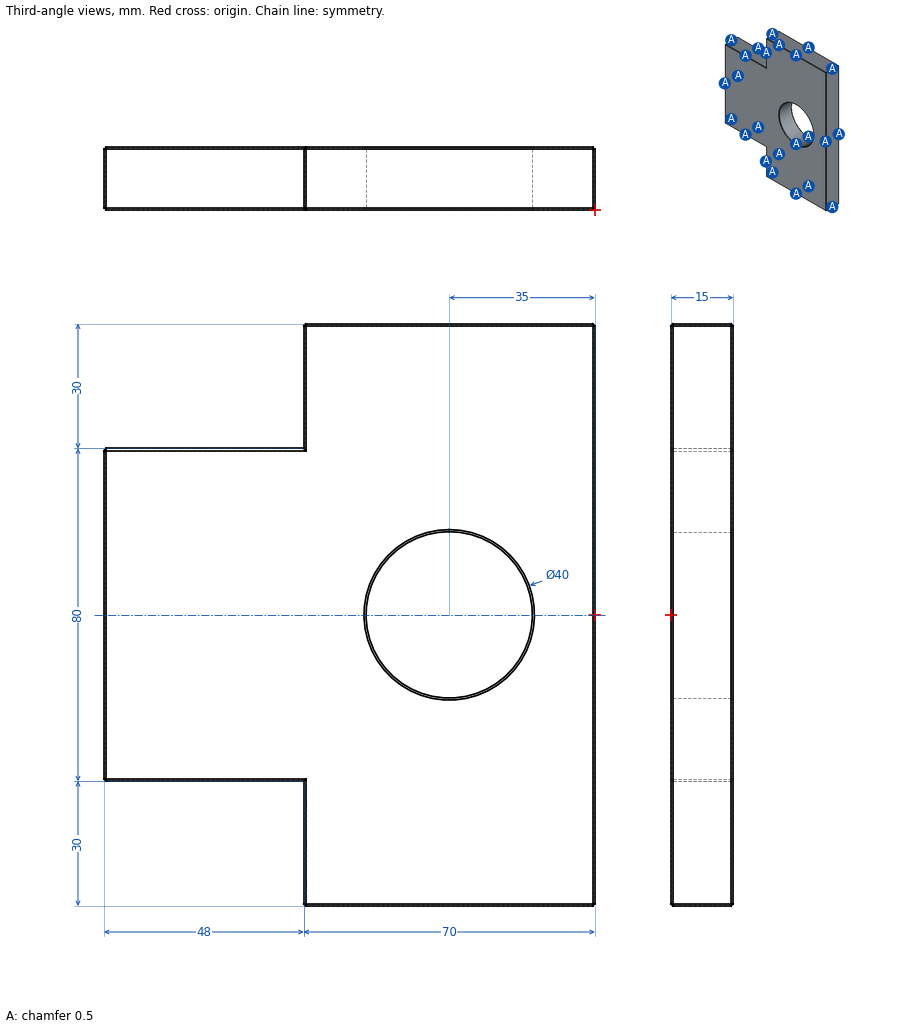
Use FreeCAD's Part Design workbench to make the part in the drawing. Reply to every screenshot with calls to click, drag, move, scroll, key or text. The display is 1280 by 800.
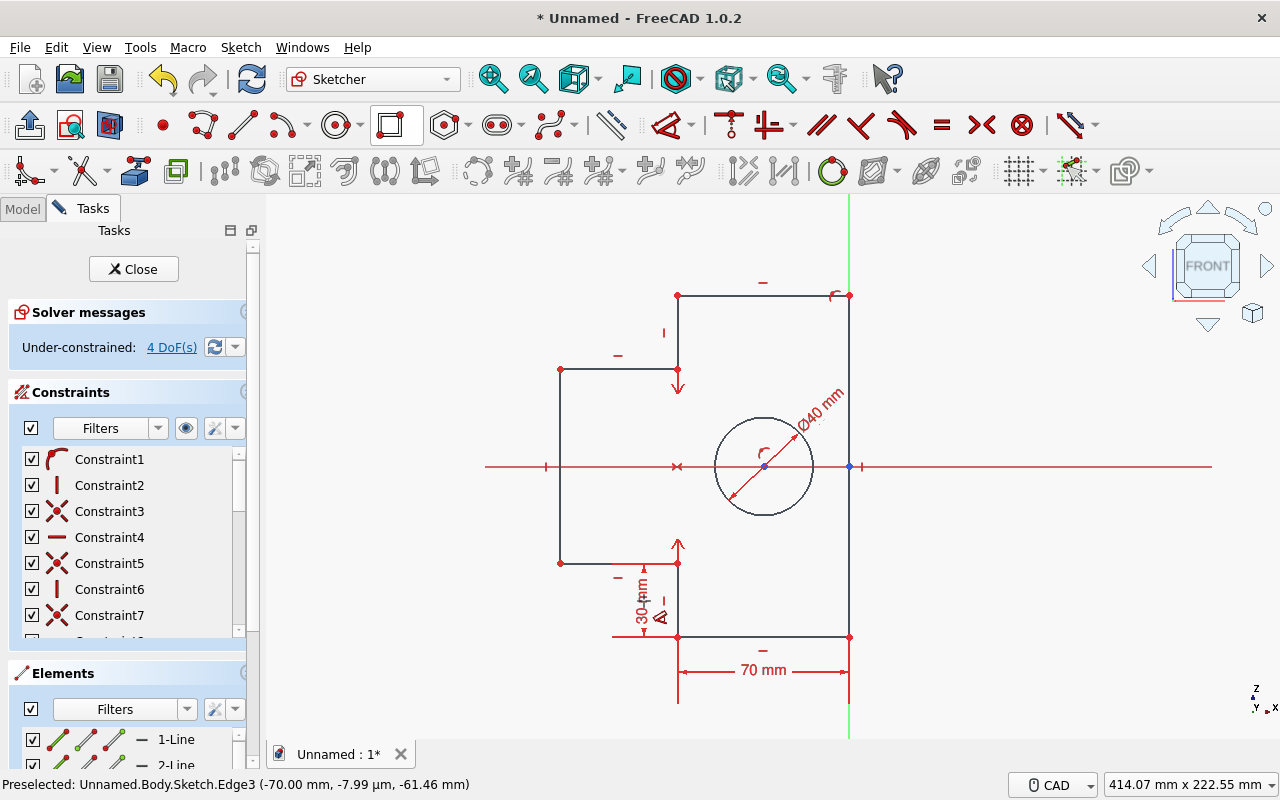
click(643, 564)
click(619, 530)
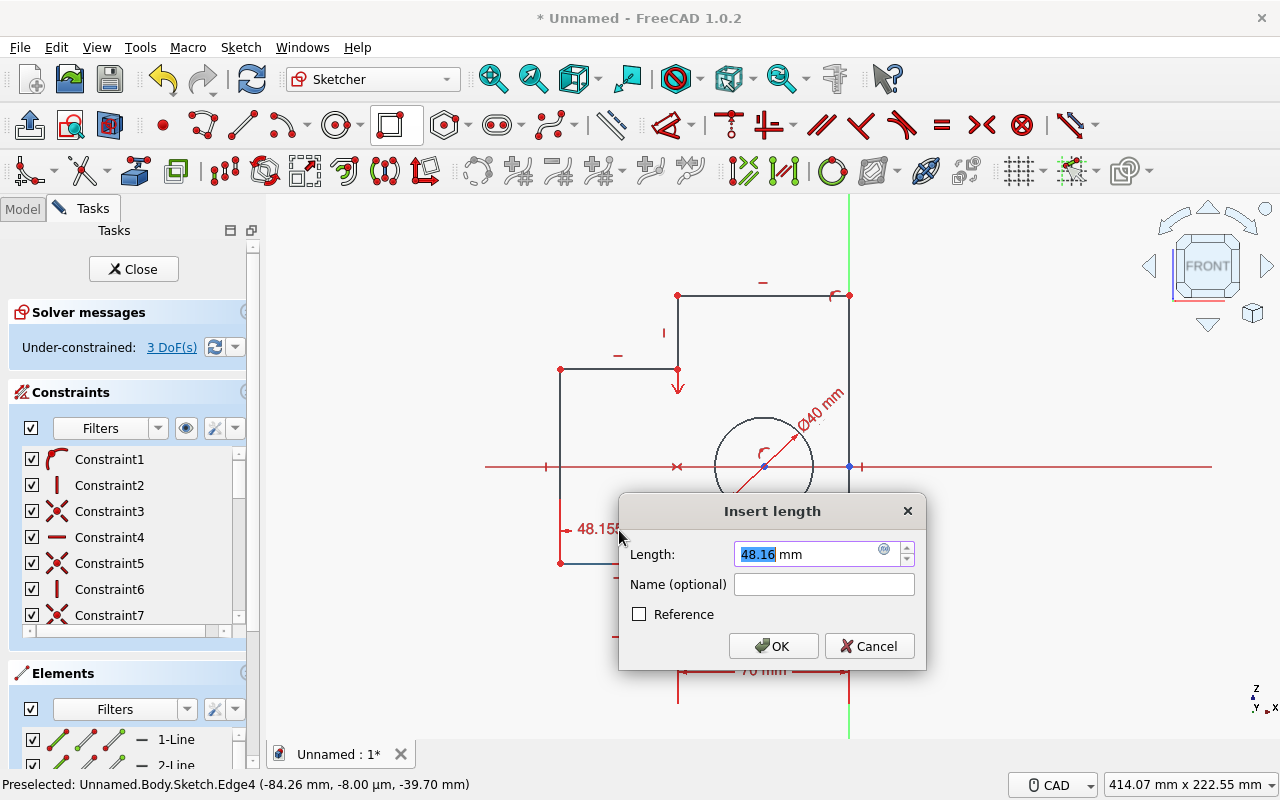
text(48)
key(Return)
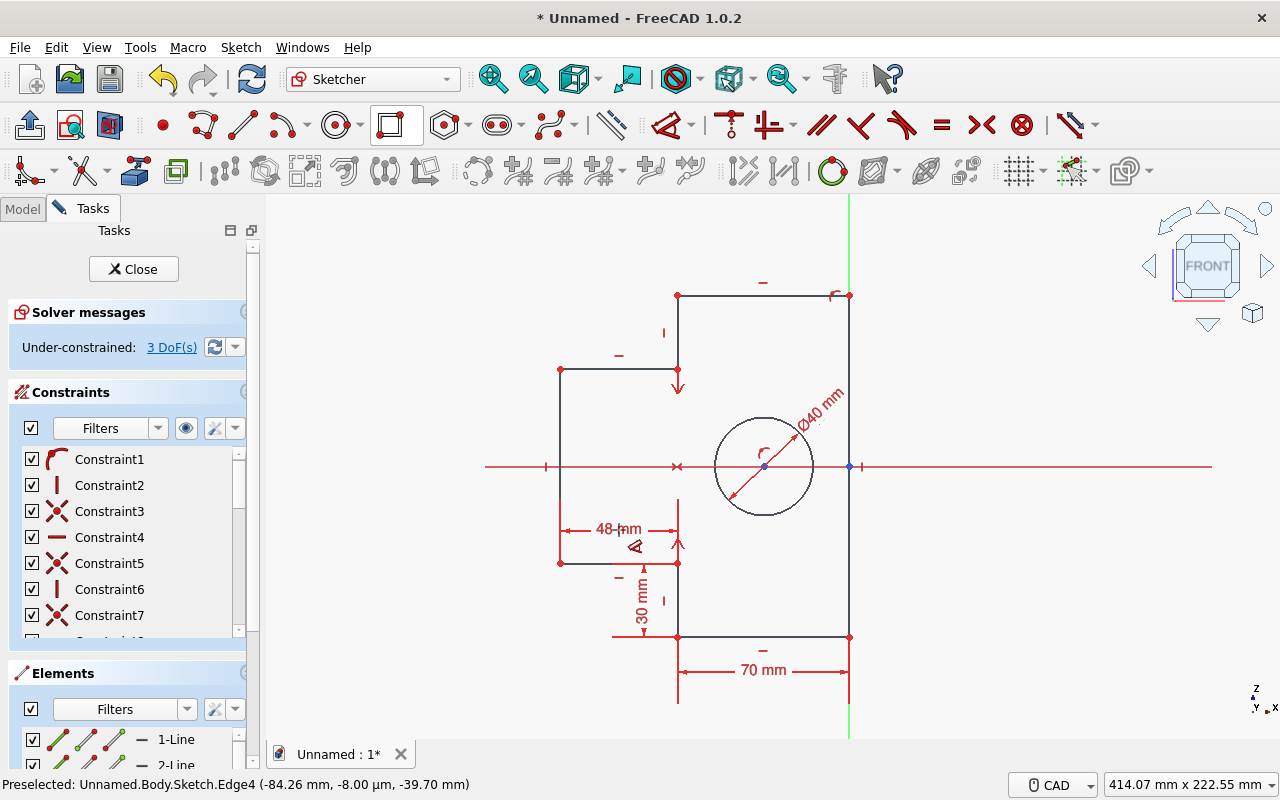
click(560, 505)
click(526, 422)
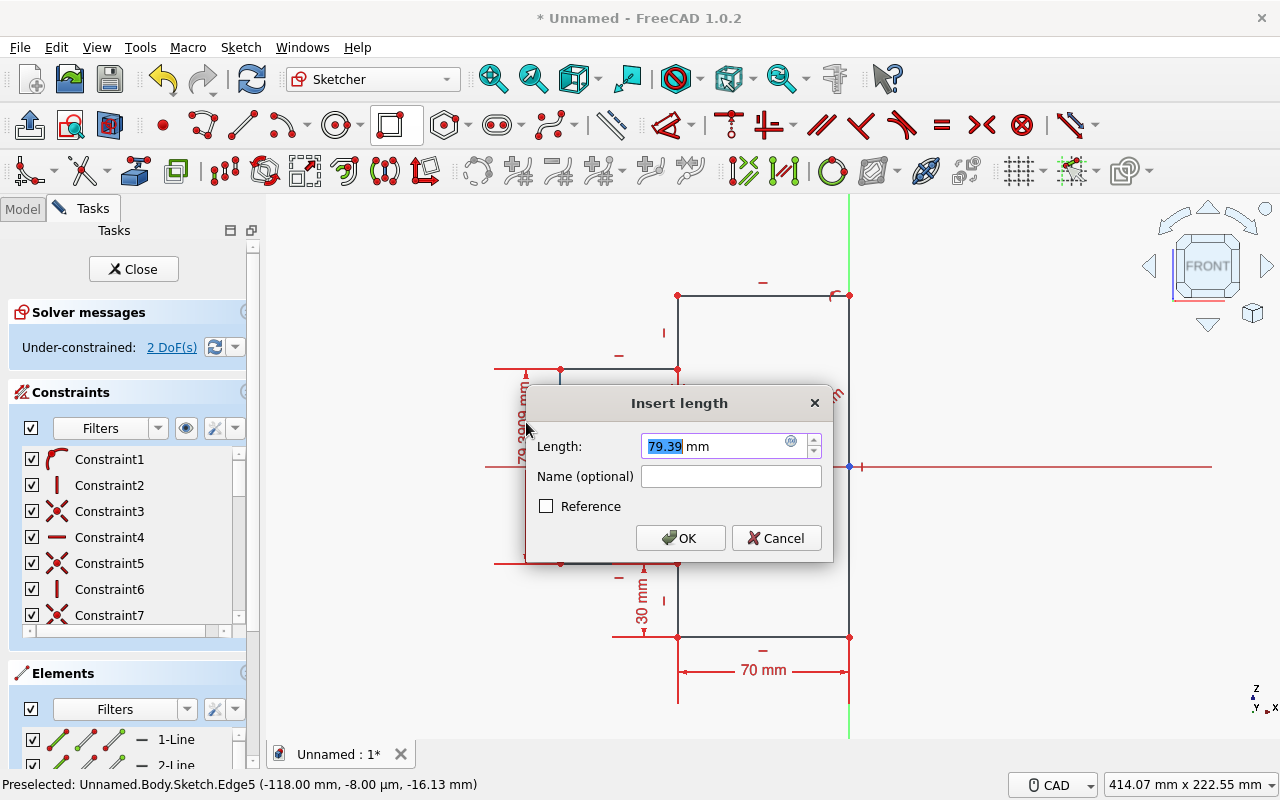
text(80)
key(Return)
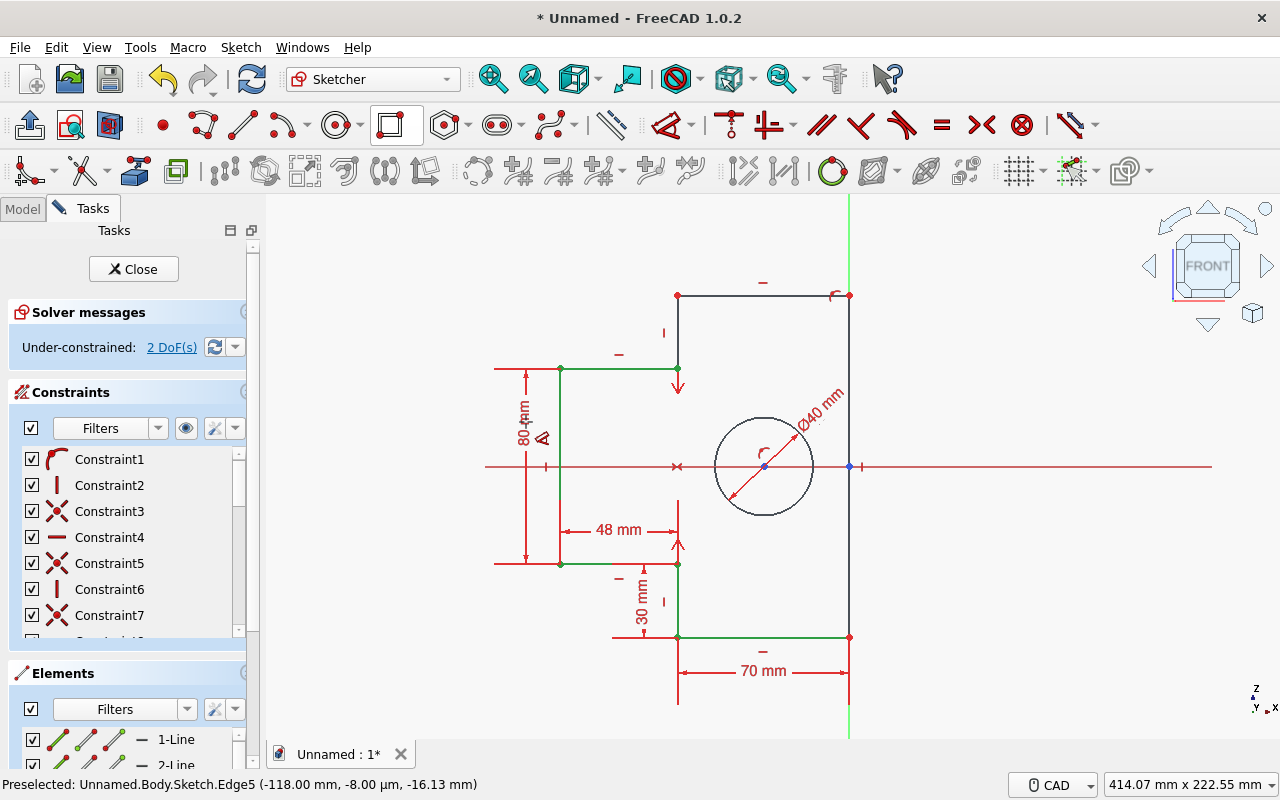
click(678, 347)
click(644, 332)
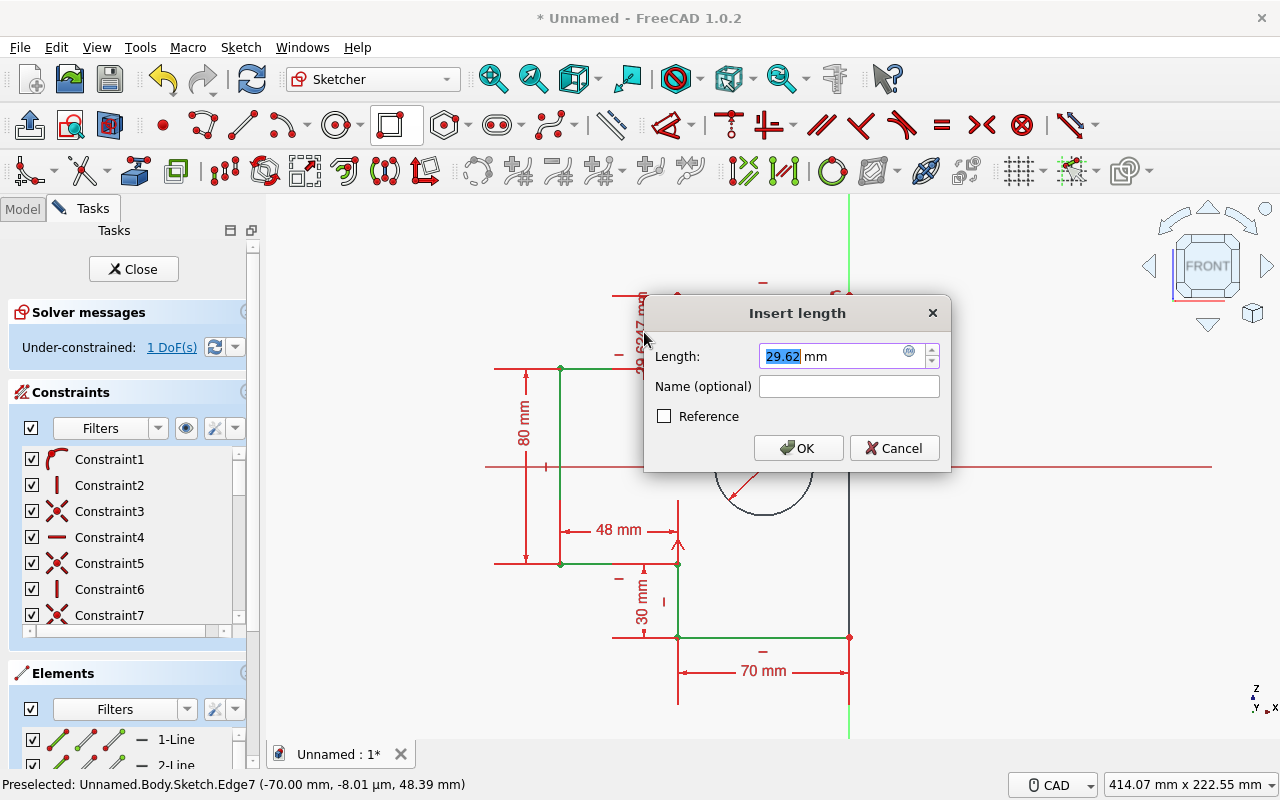
text(30)
key(Return)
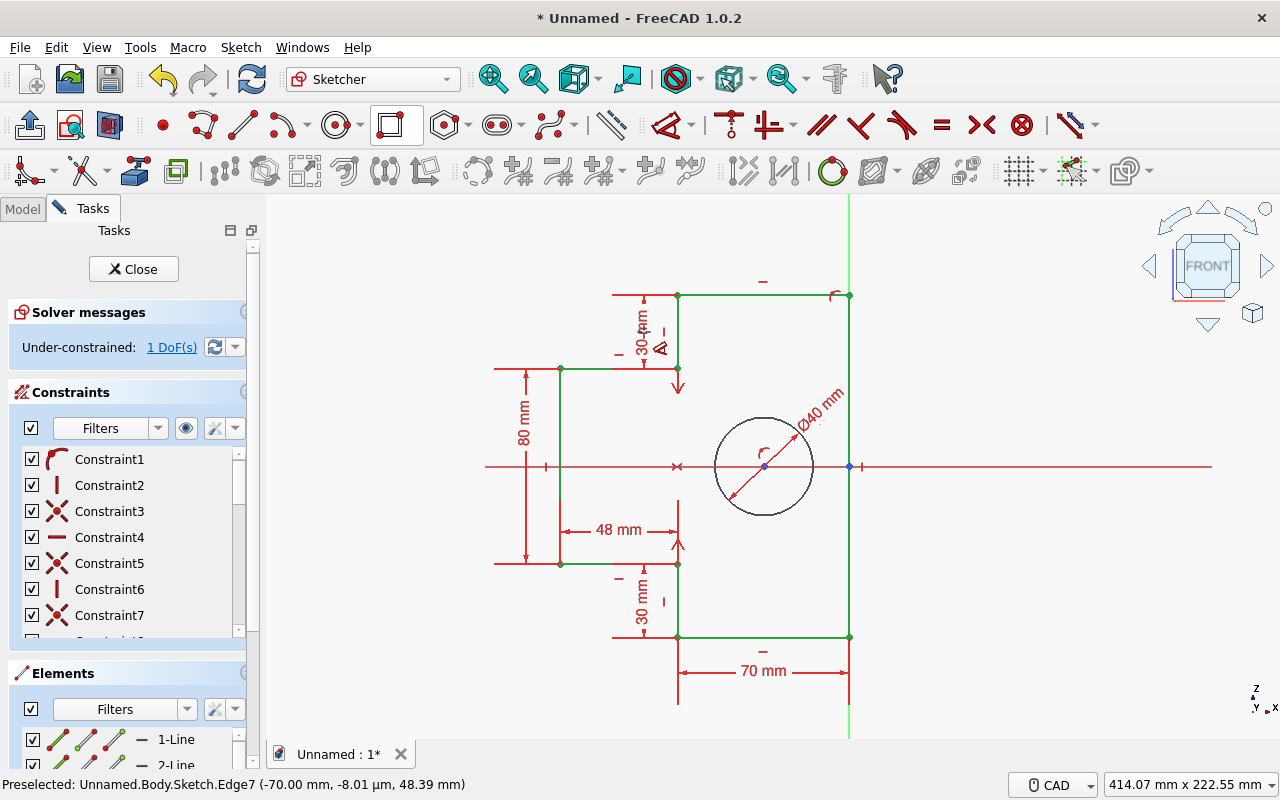
click(764, 466)
click(826, 500)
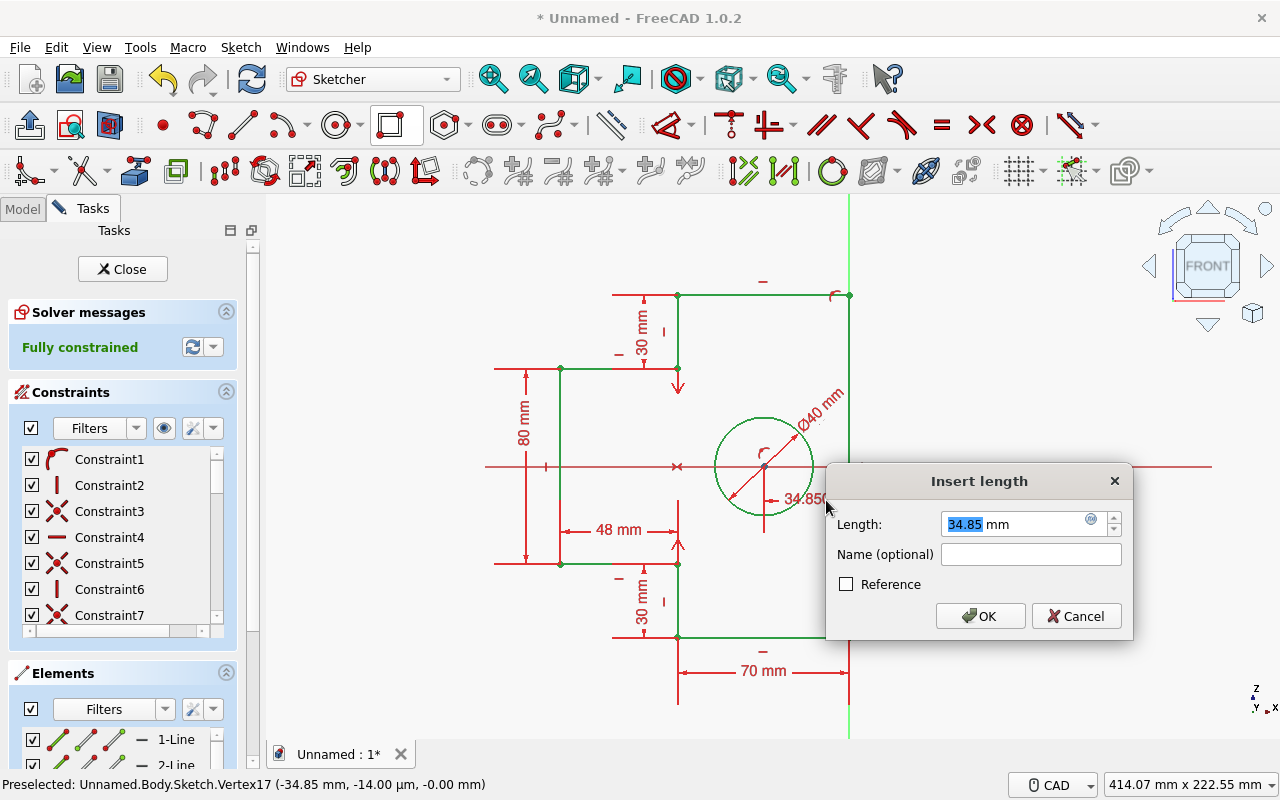
text(35)
key(Return)
key(Escape)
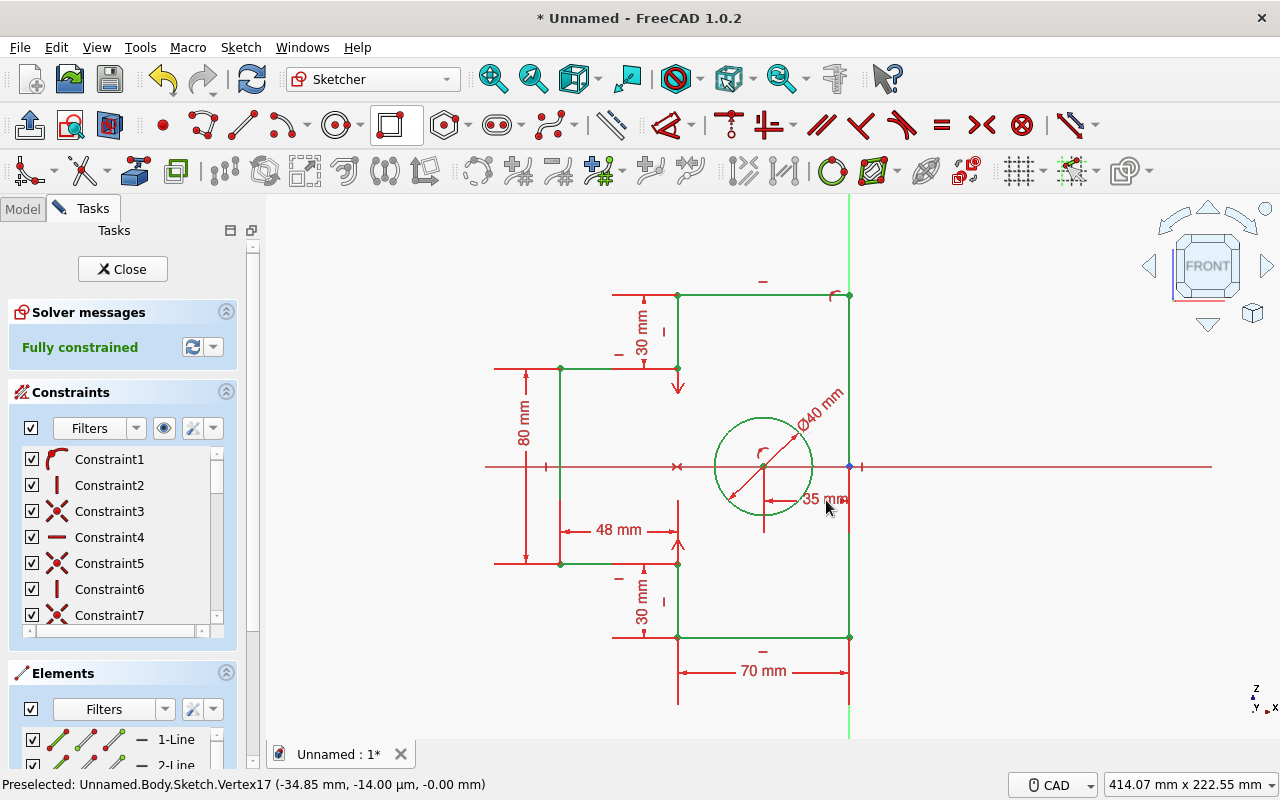
click(123, 269)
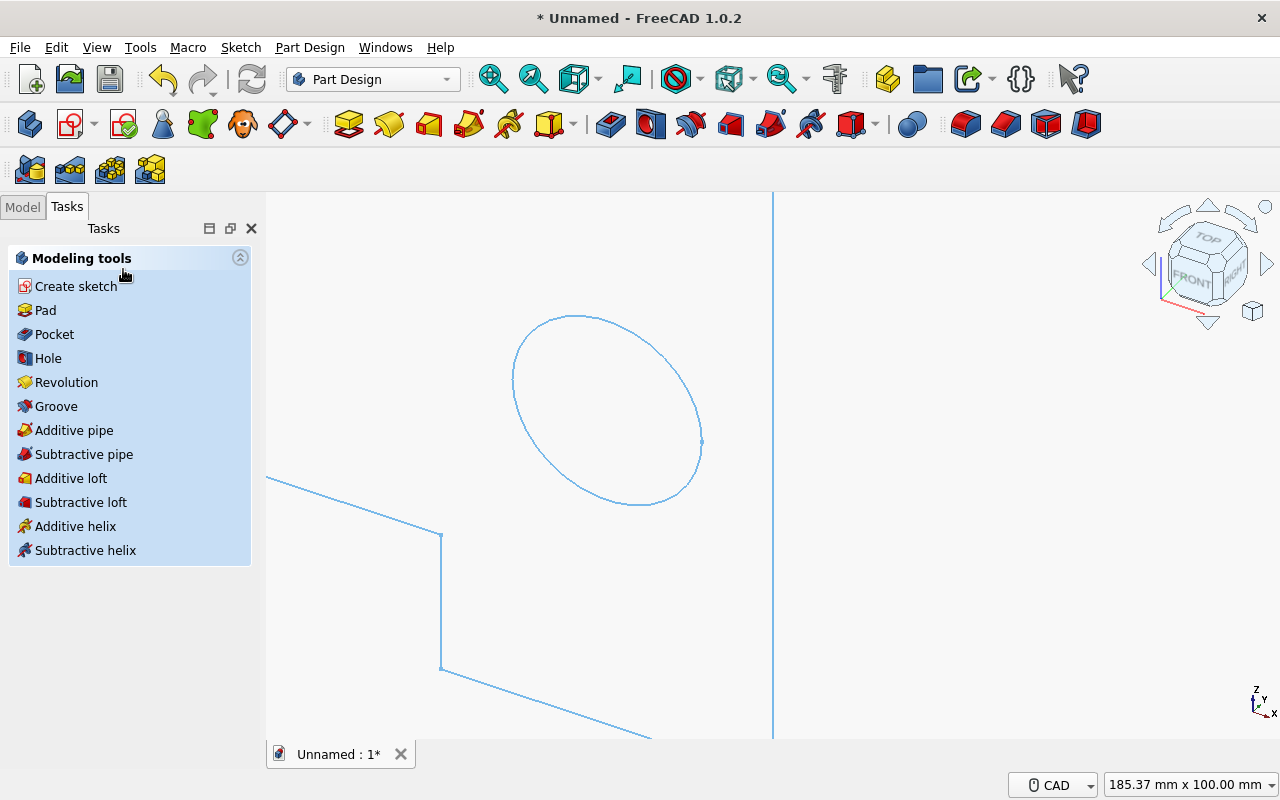
click(350, 124)